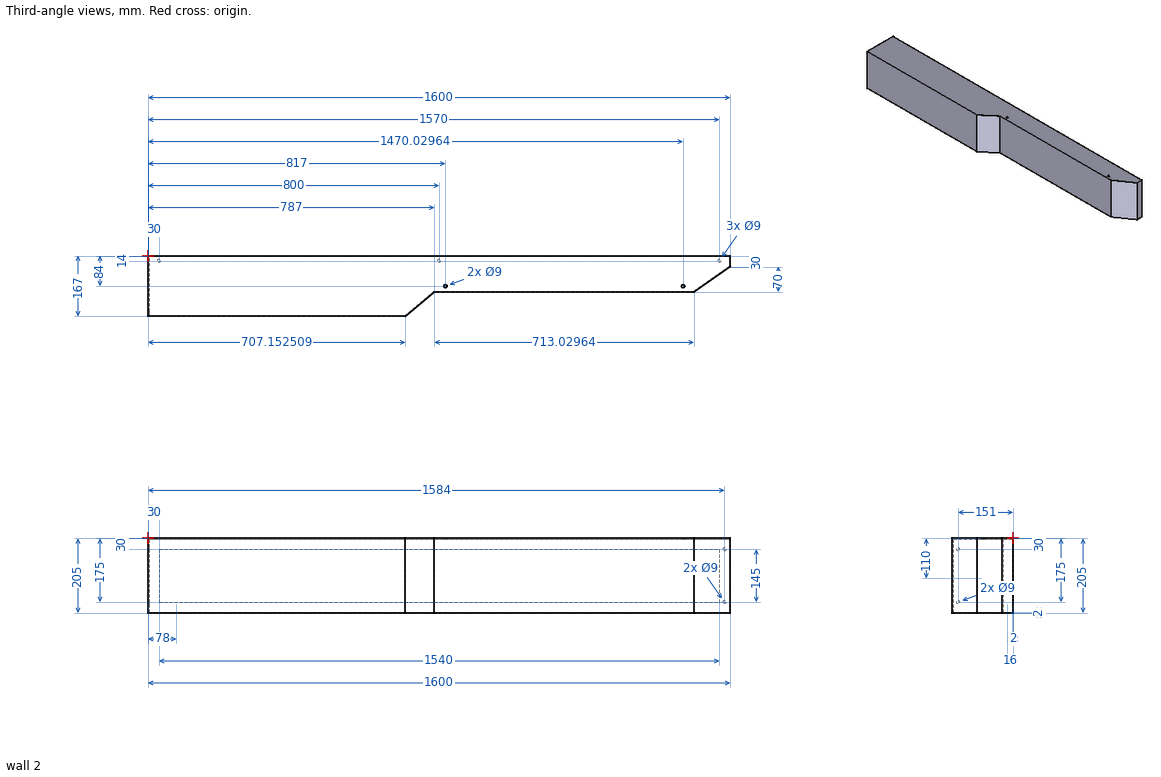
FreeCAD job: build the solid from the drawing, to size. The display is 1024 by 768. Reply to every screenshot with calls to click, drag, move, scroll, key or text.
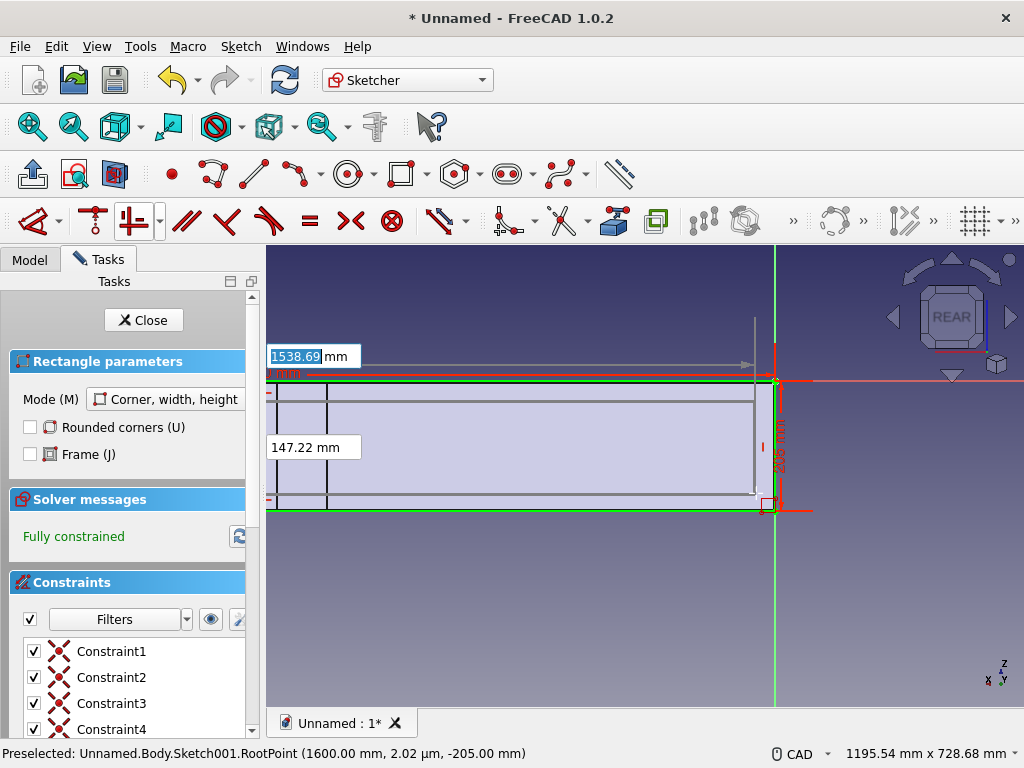
click(756, 492)
key(Escape)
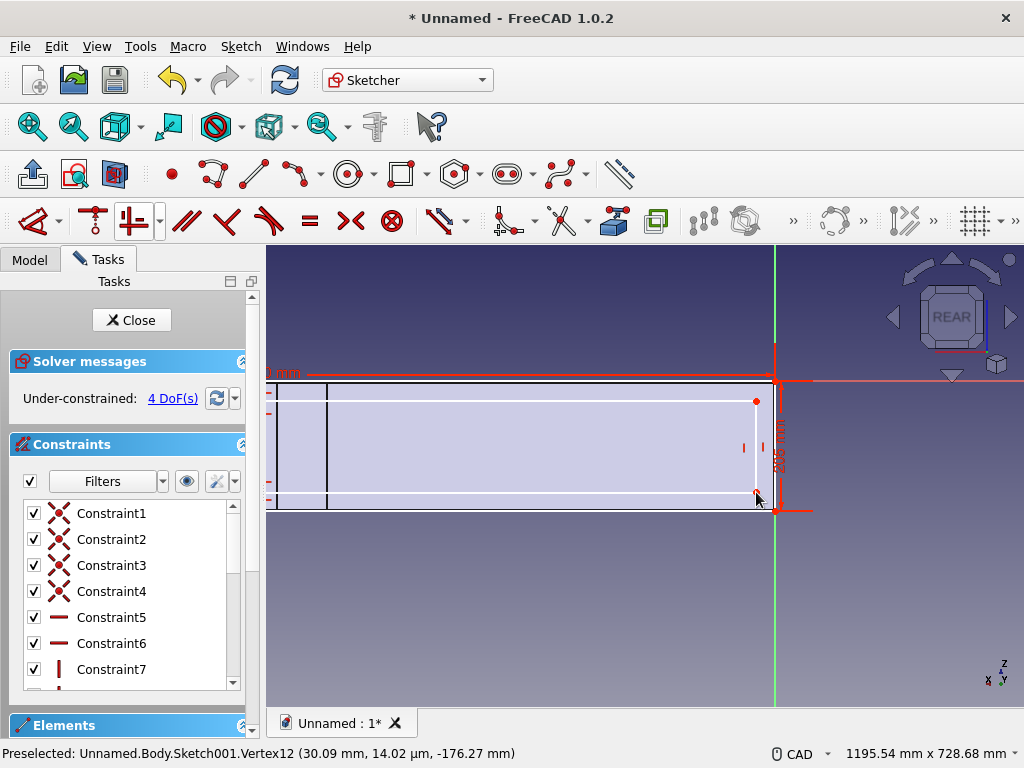
click(32, 222)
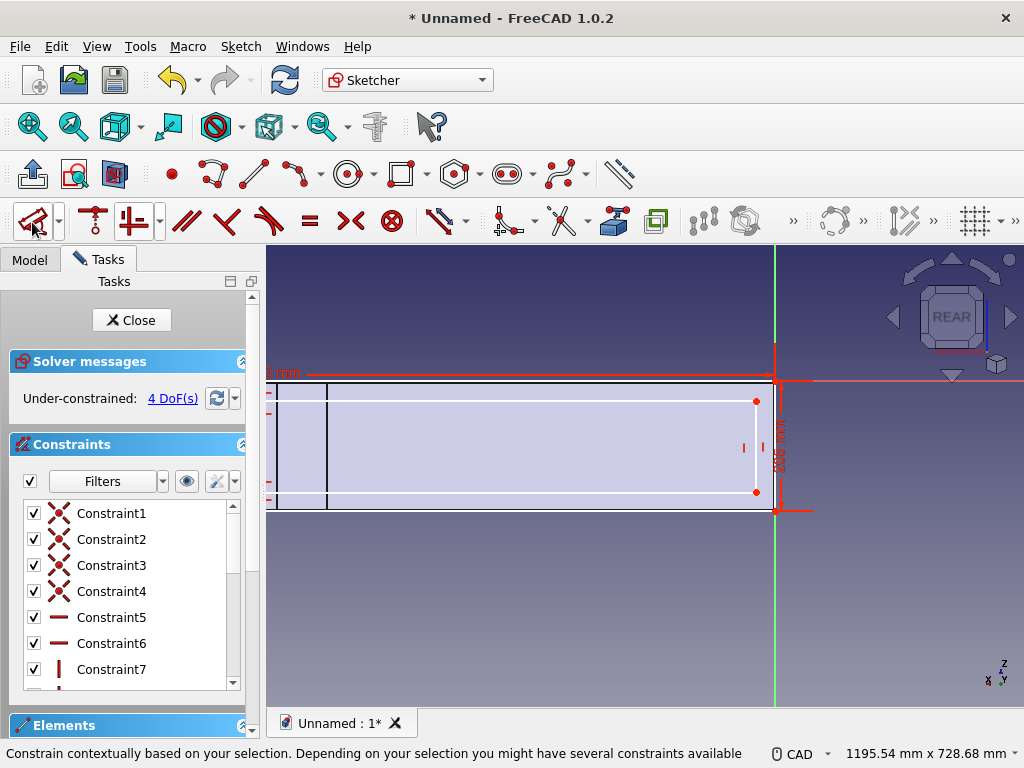
scroll(756, 493, down, 5)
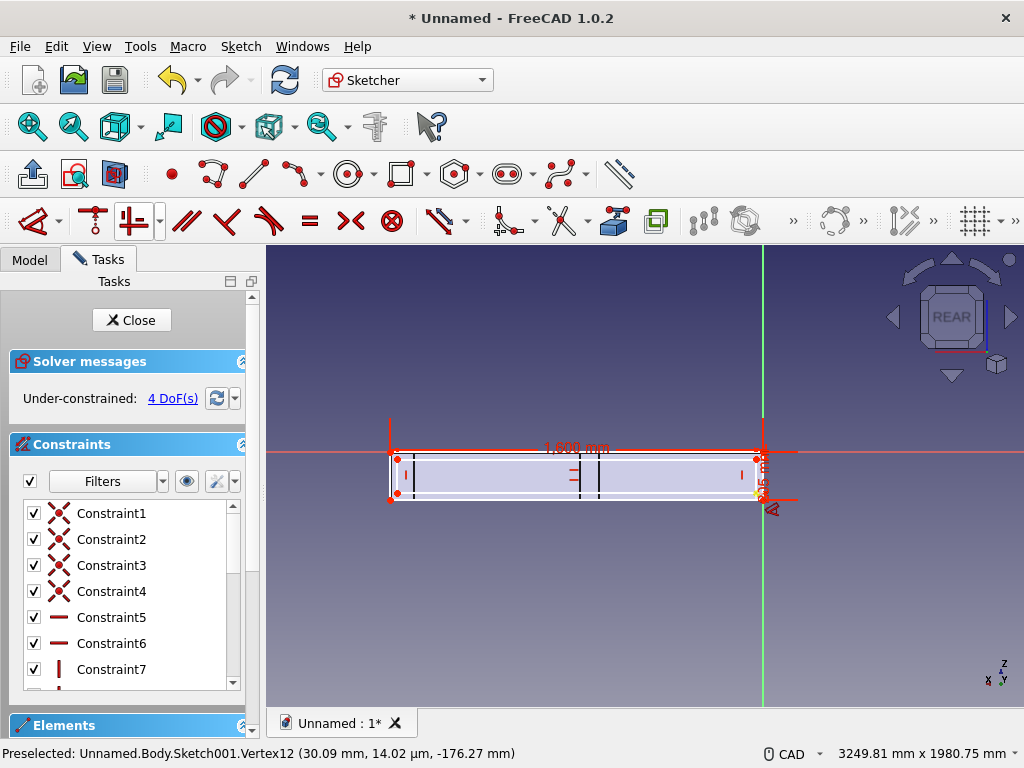
scroll(397, 470, up, 4)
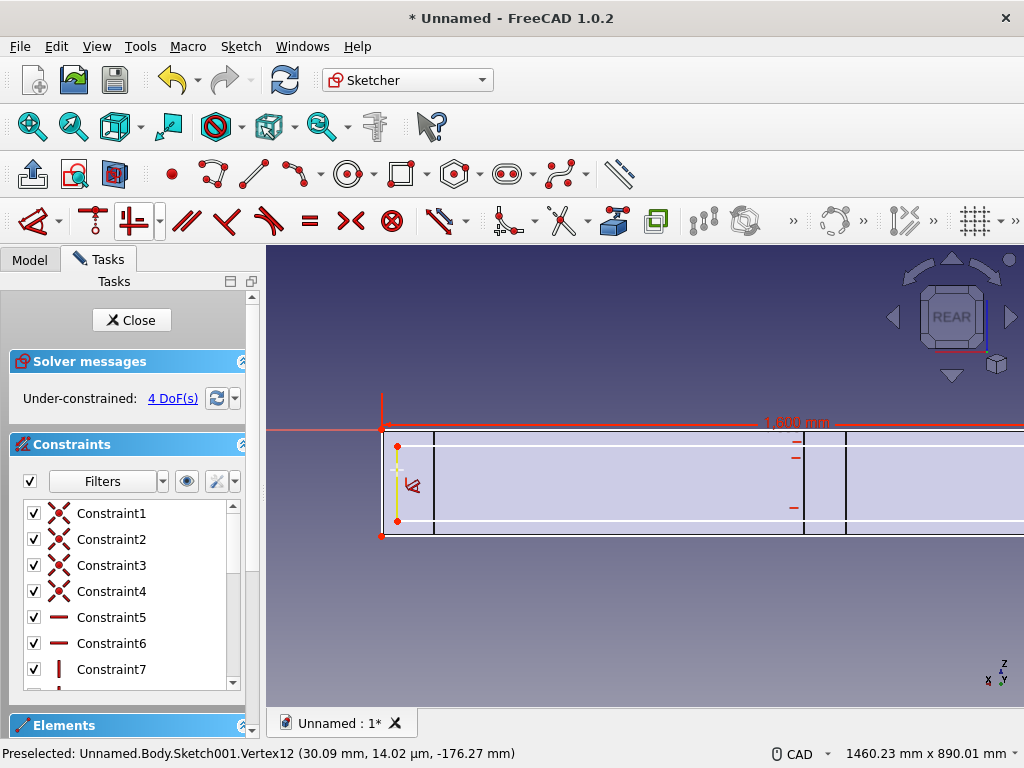
click(397, 469)
click(363, 484)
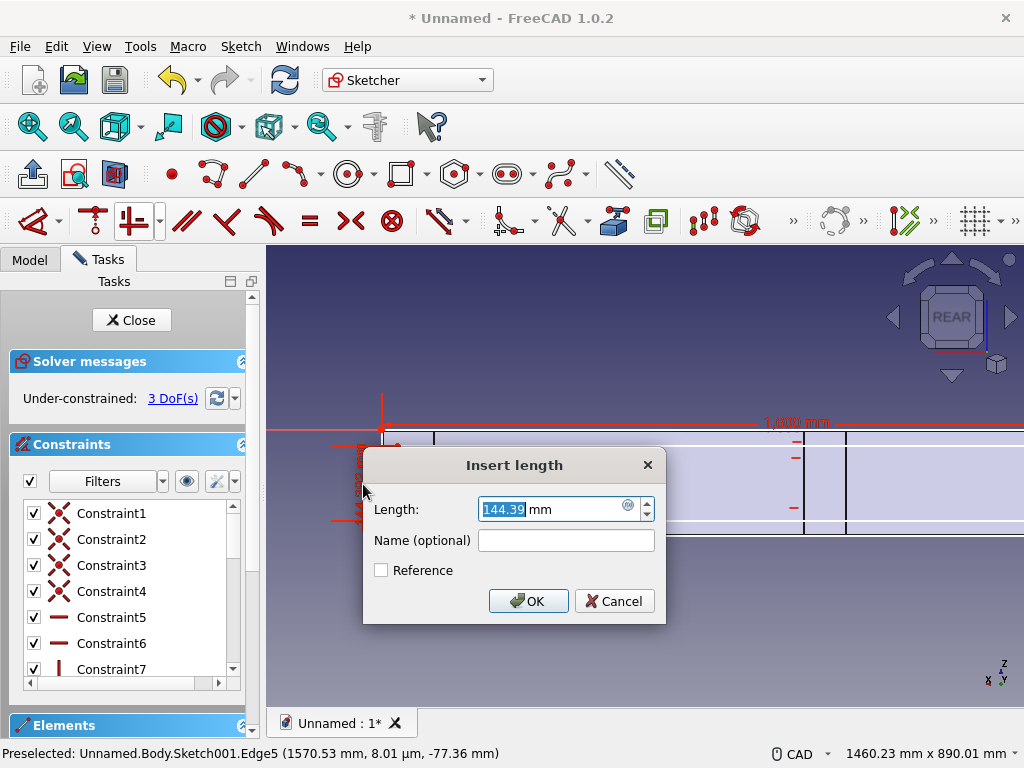
text(145)
key(Return)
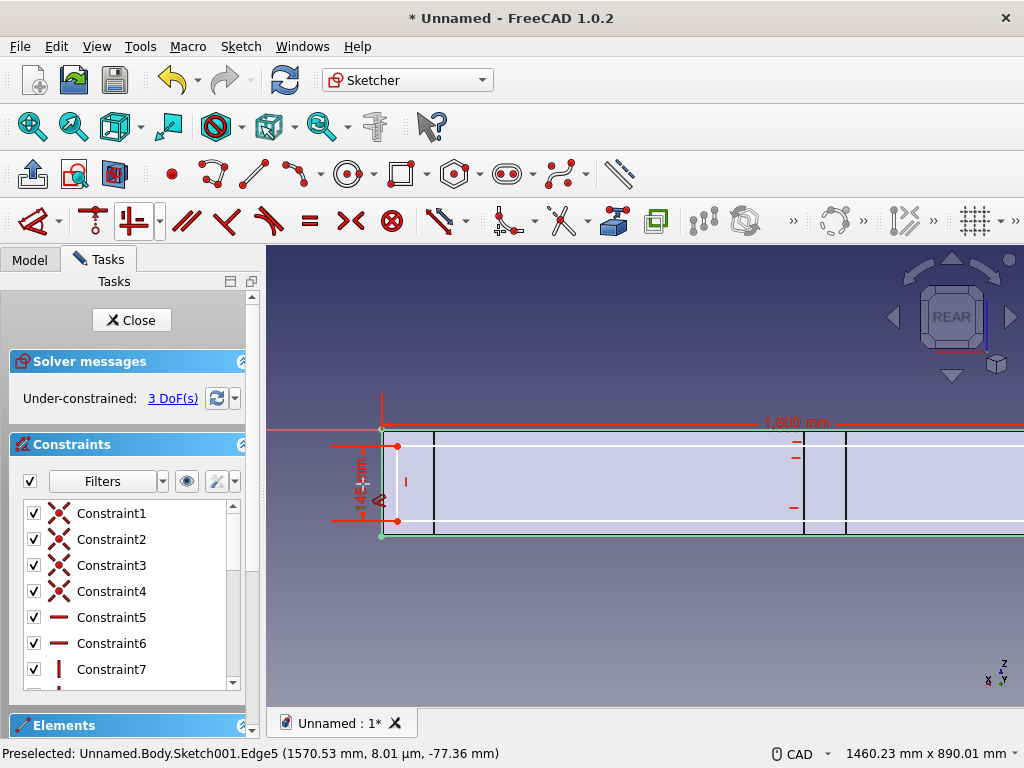
scroll(397, 446, up, 5)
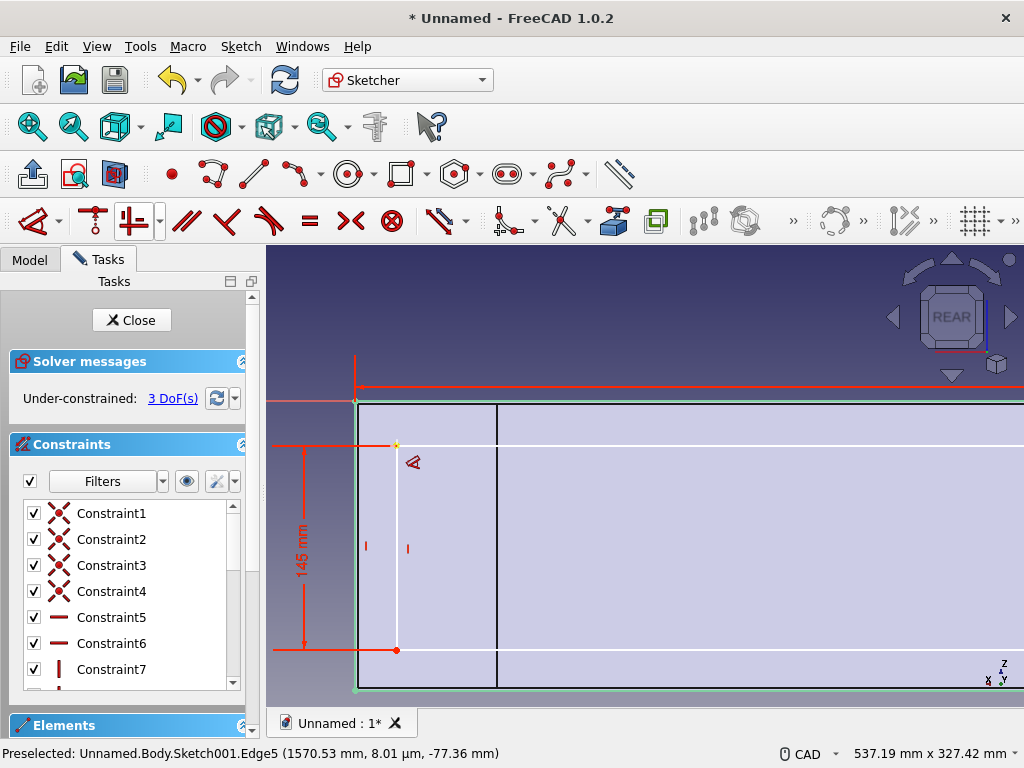
click(397, 446)
click(339, 424)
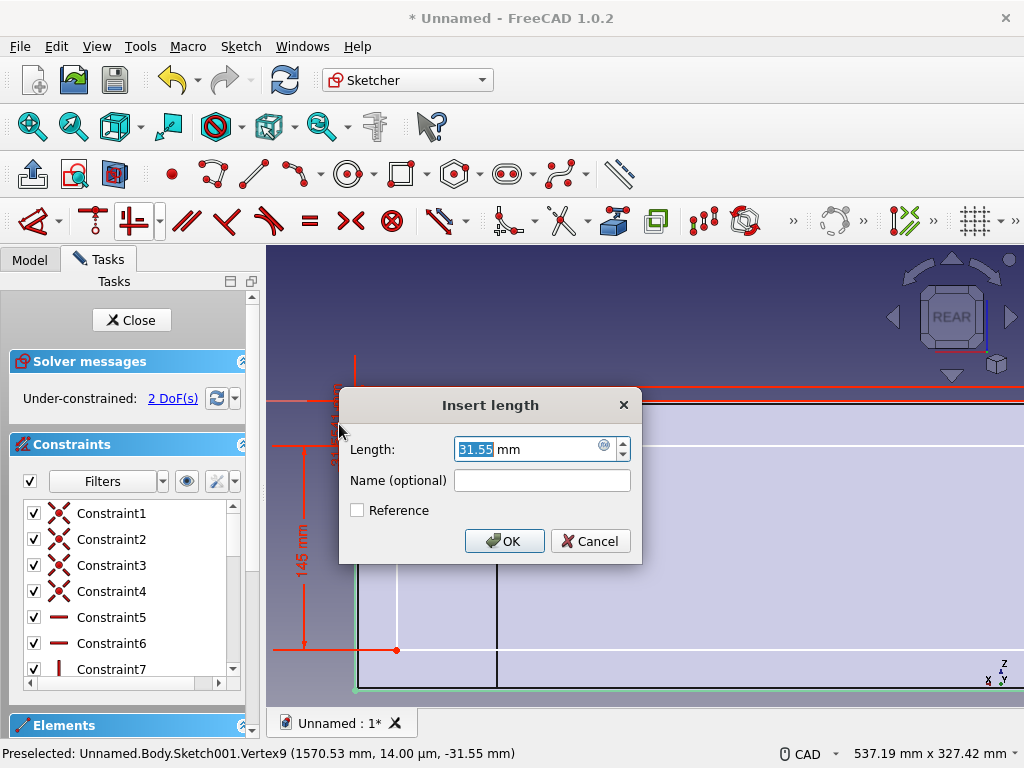
text(30)
key(Return)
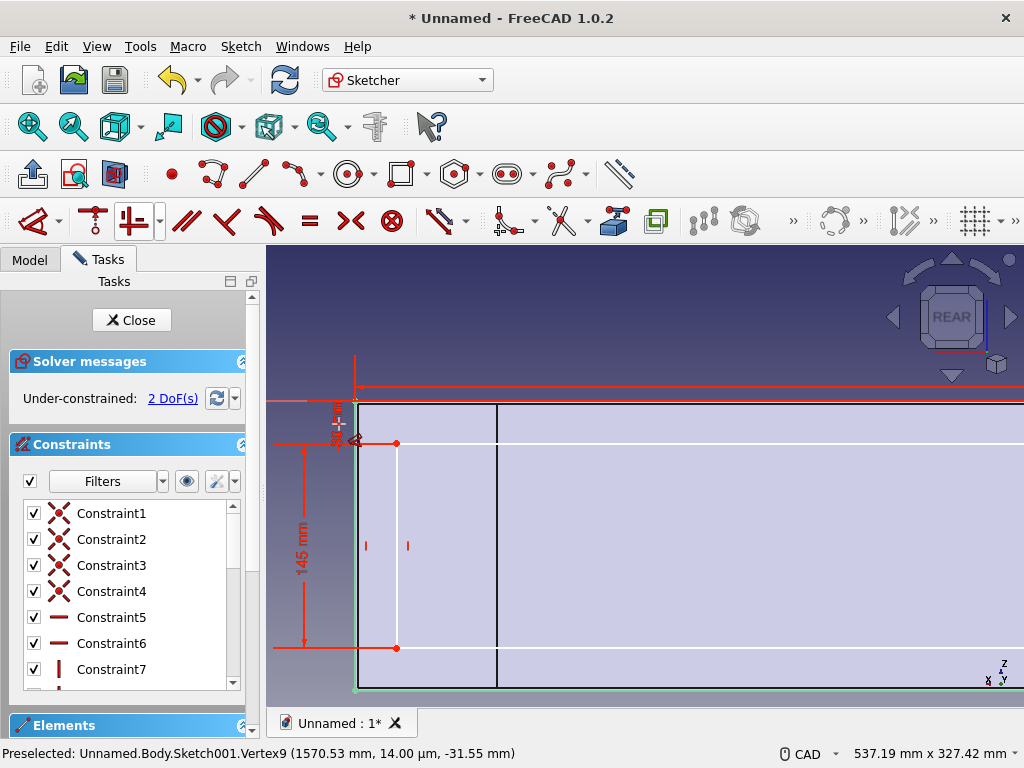
scroll(397, 462, down, 9)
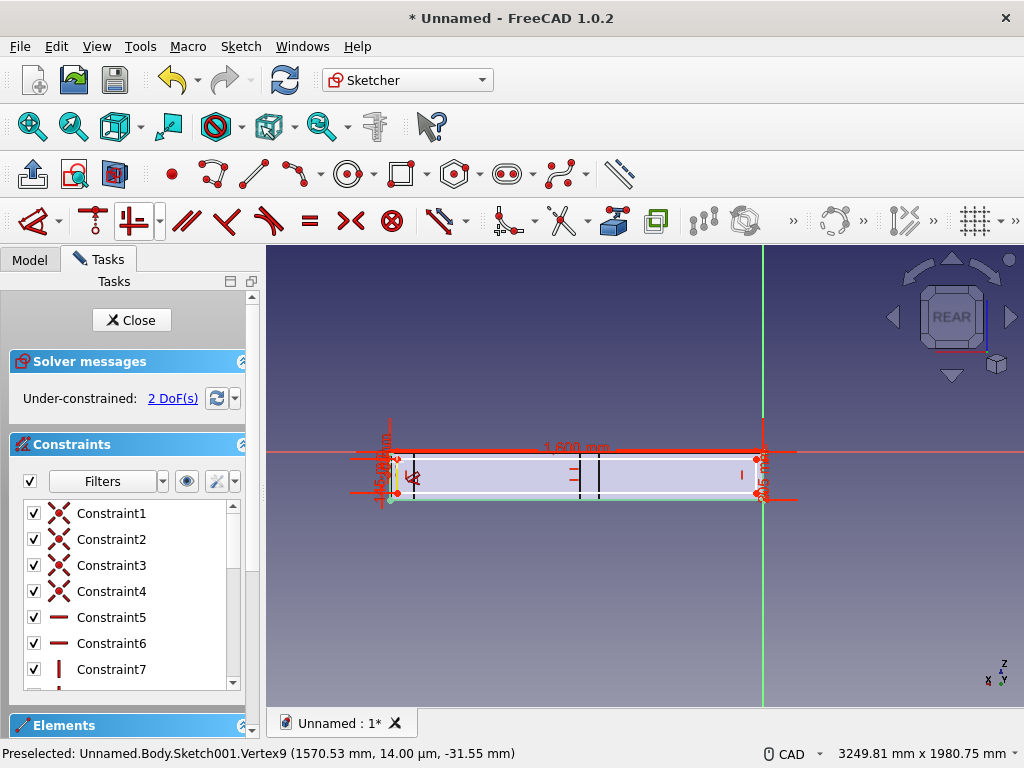
scroll(756, 493, up, 9)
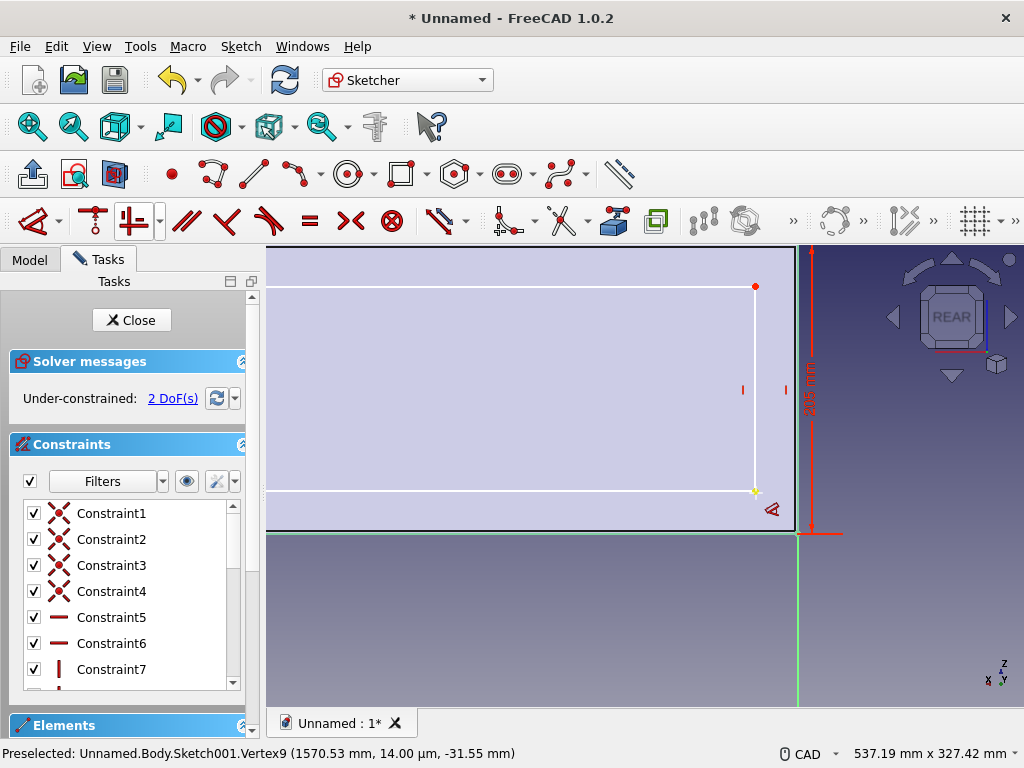
click(755, 491)
click(776, 549)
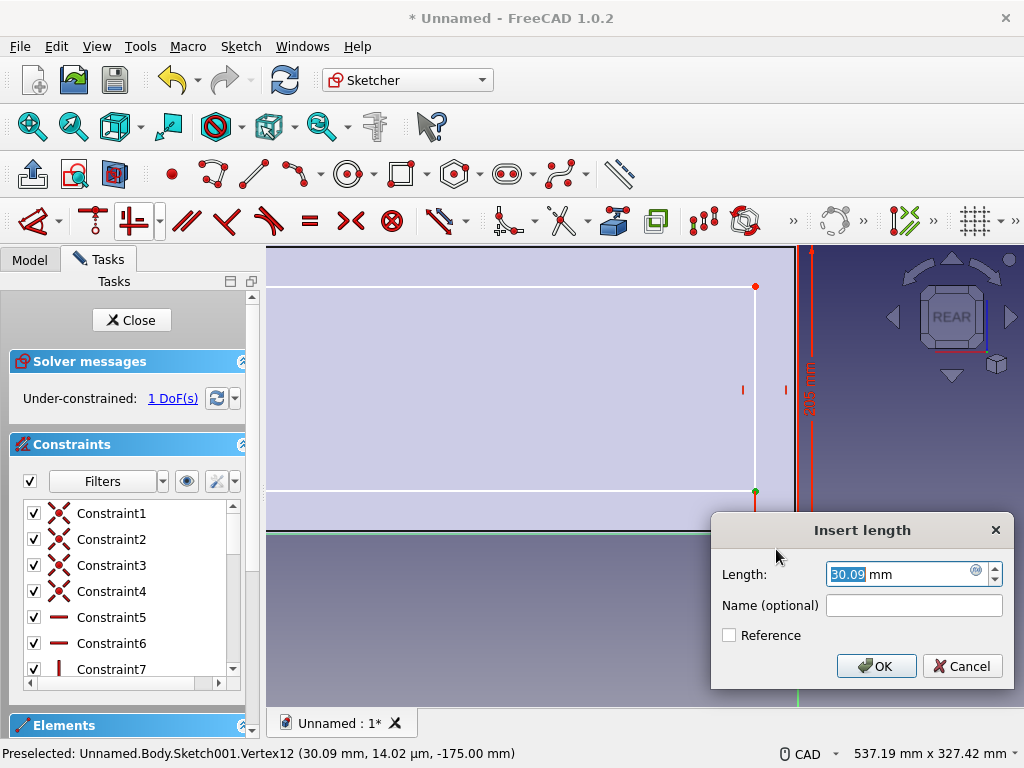
text(30)
key(Return)